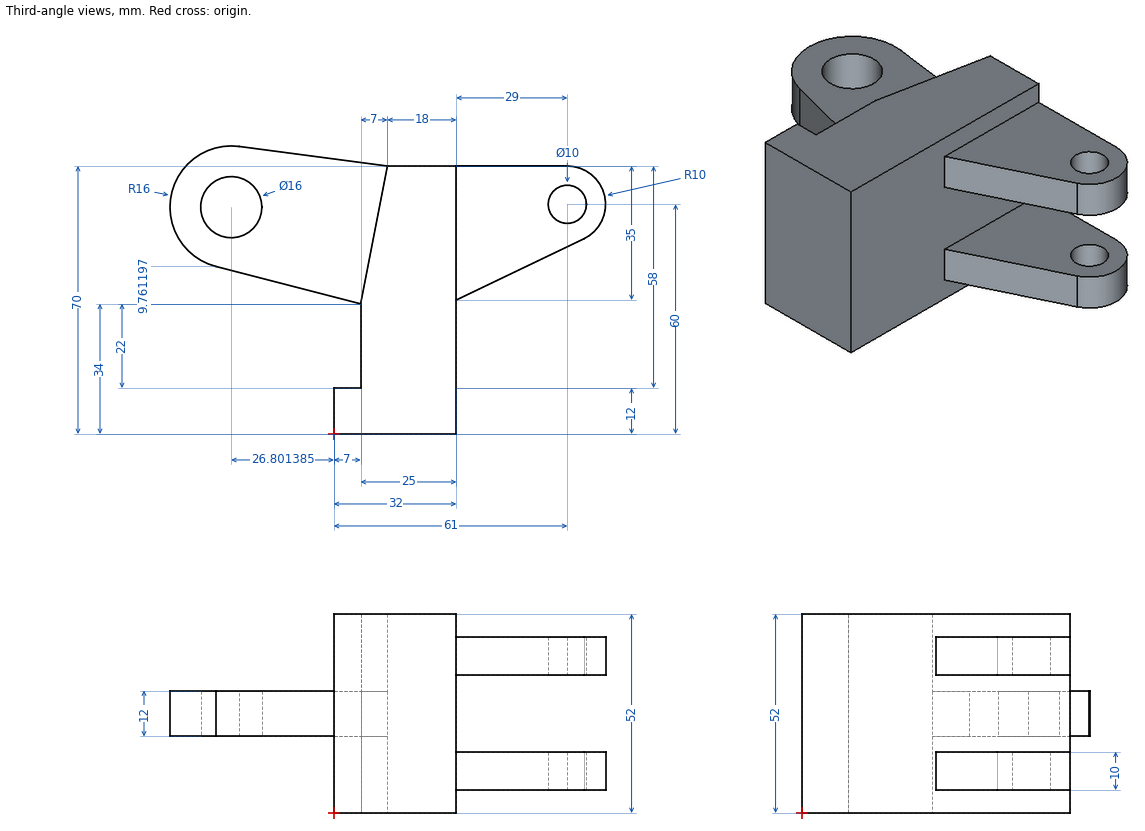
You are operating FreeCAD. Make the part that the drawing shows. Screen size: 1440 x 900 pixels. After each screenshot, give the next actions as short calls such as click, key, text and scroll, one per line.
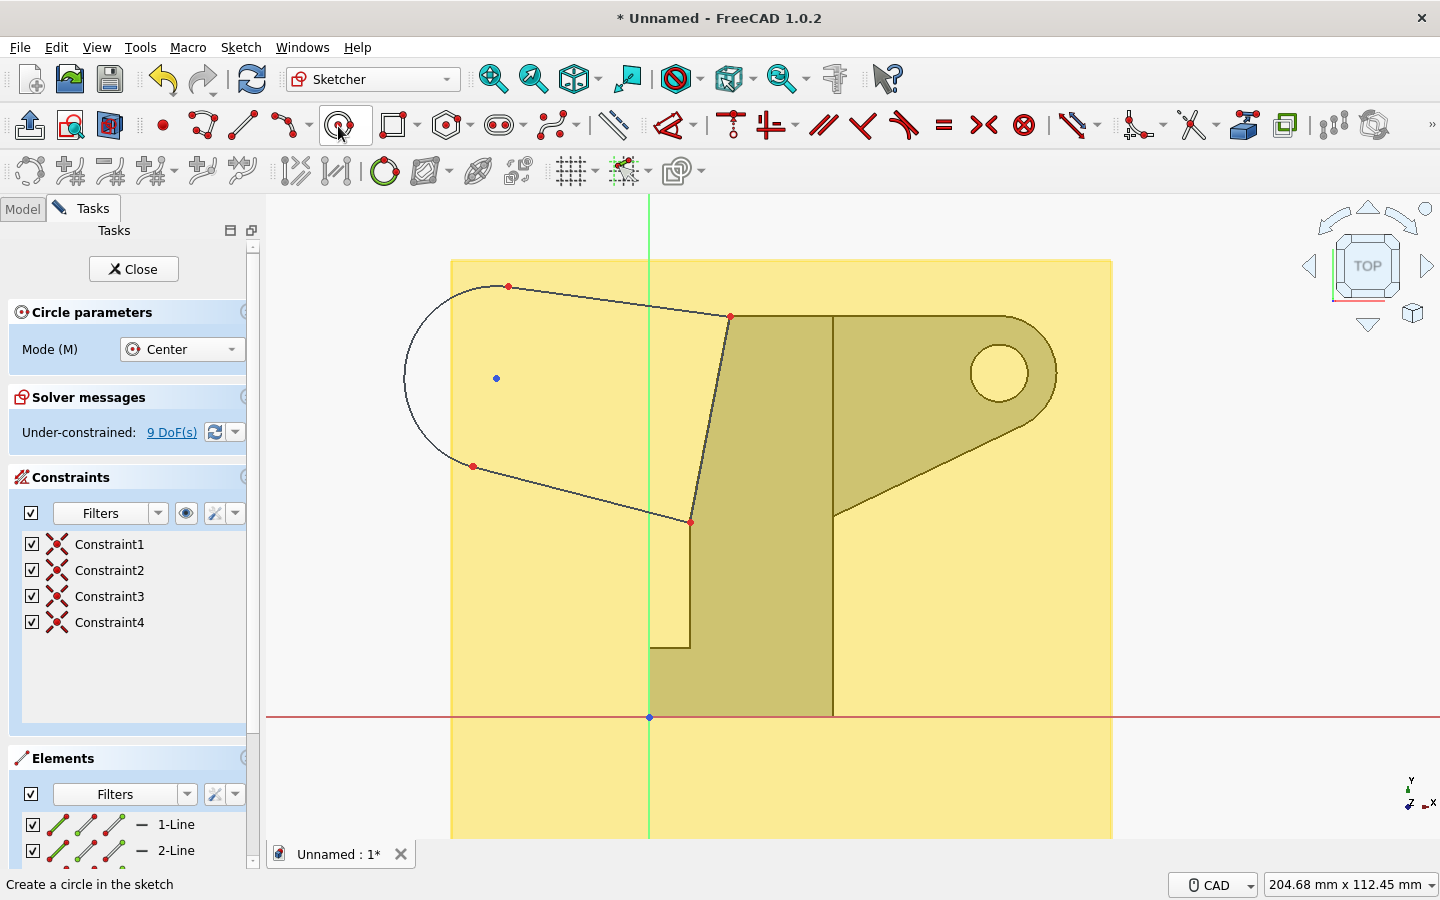
click(496, 377)
move(528, 345)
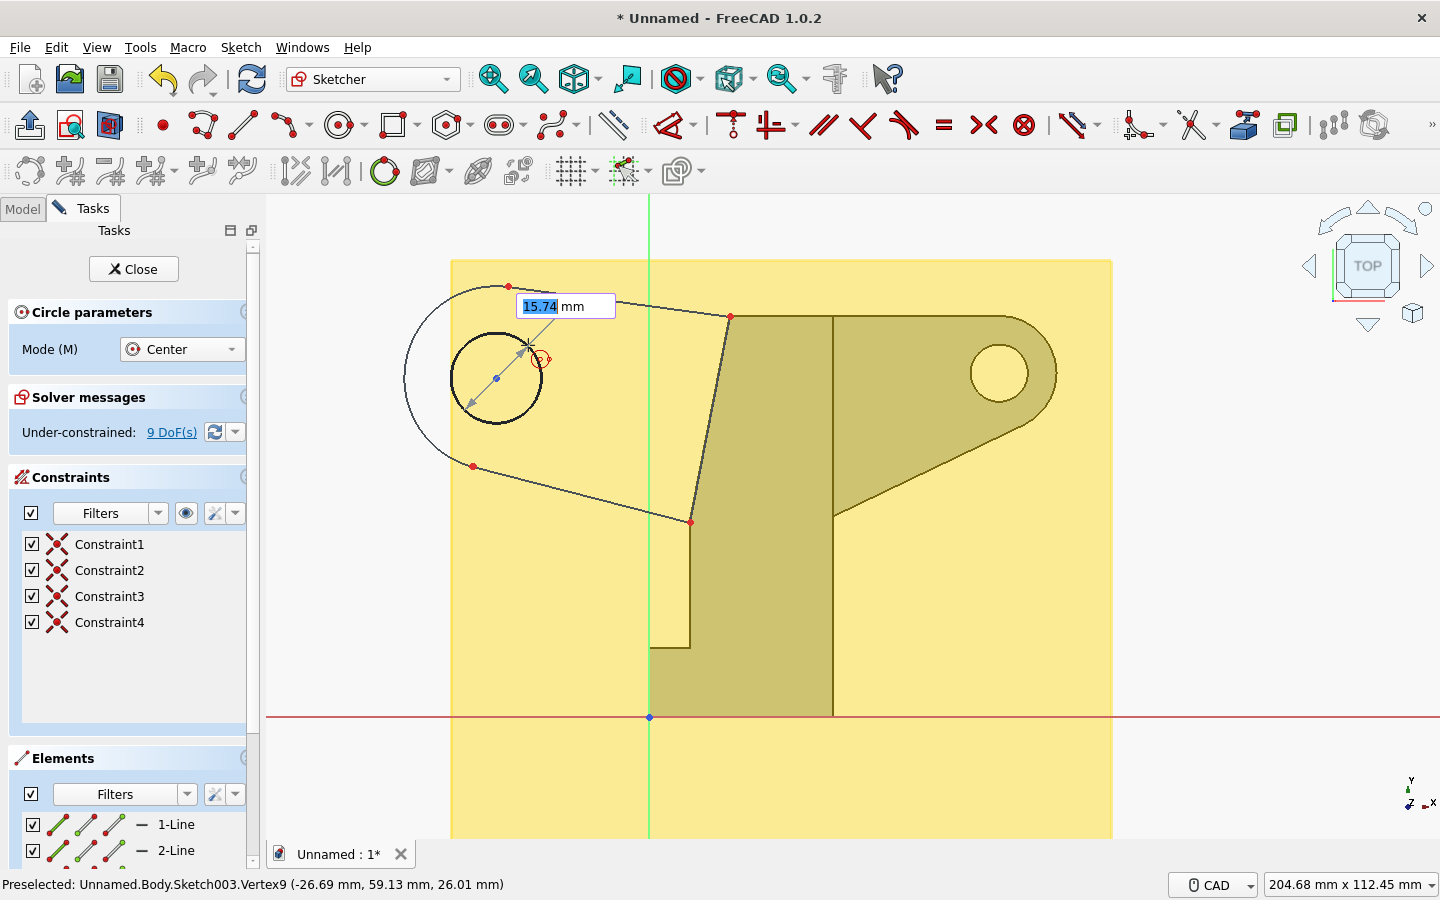
text(16)
key(Return)
key(Escape)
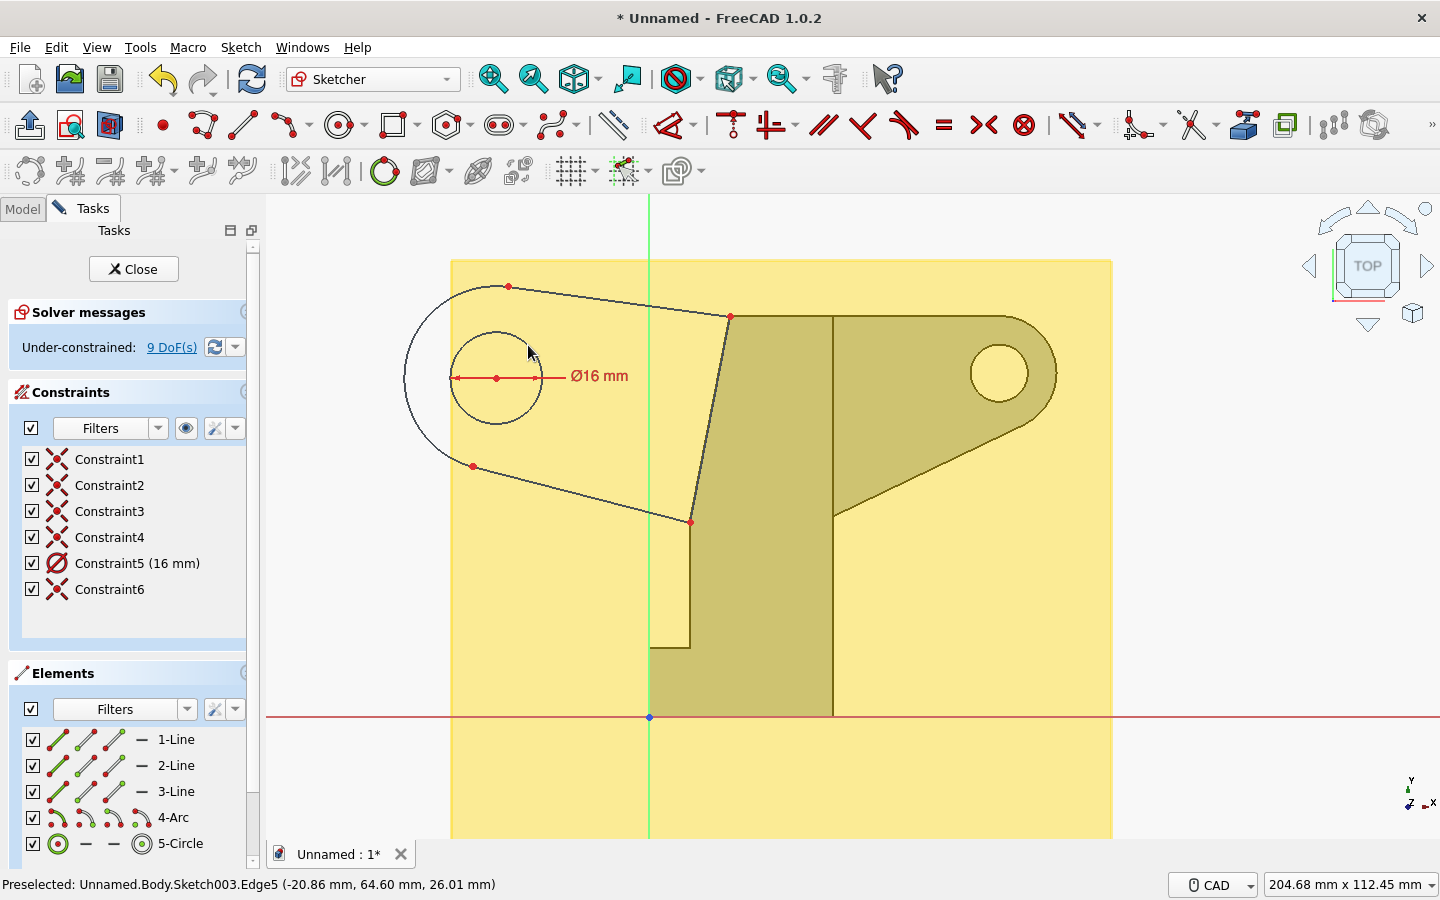
click(538, 484)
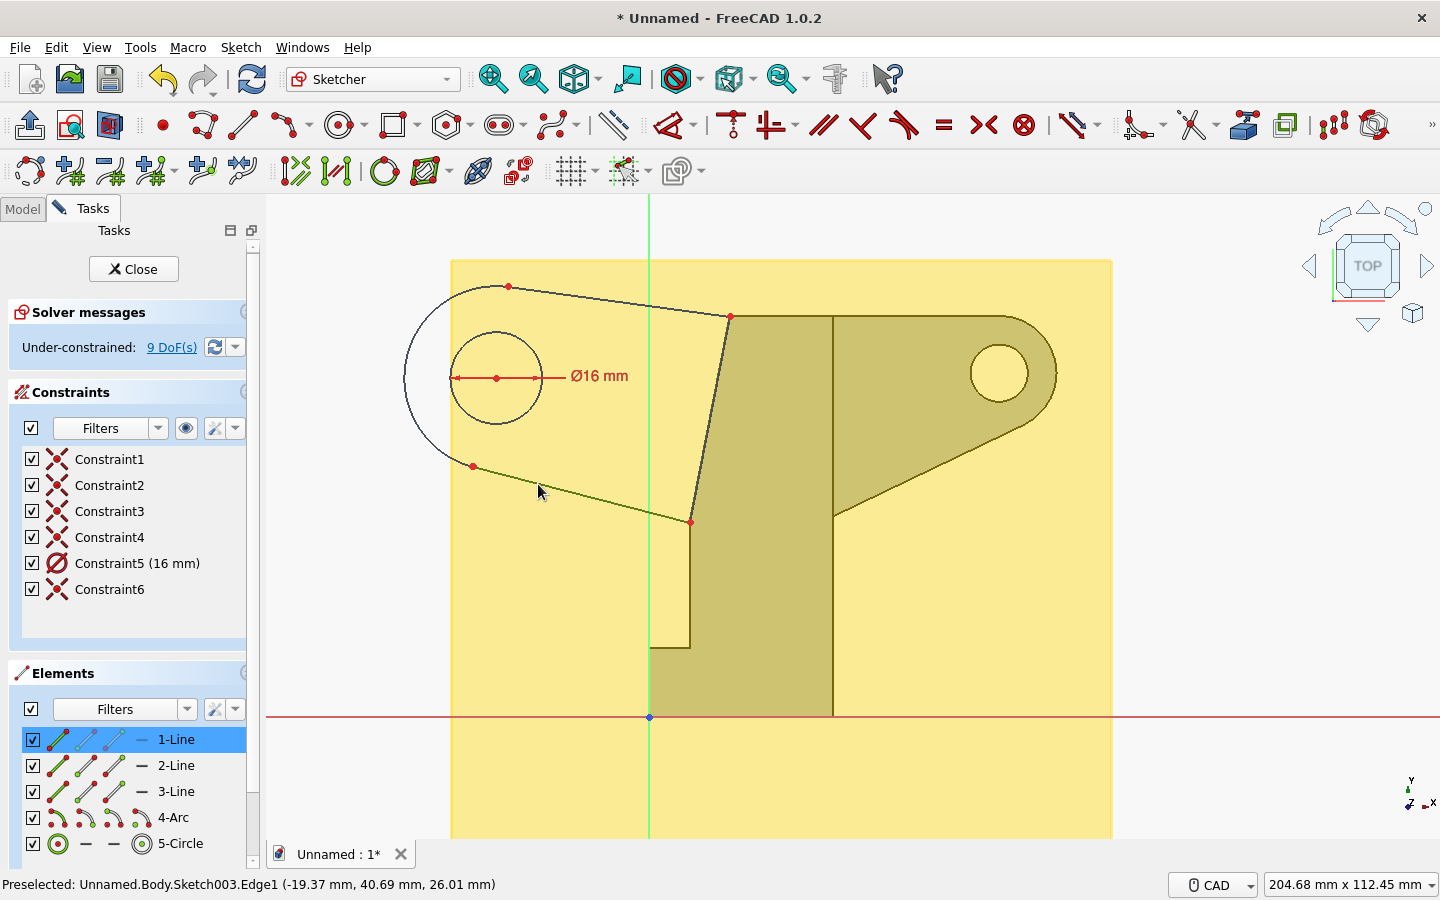
click(432, 313)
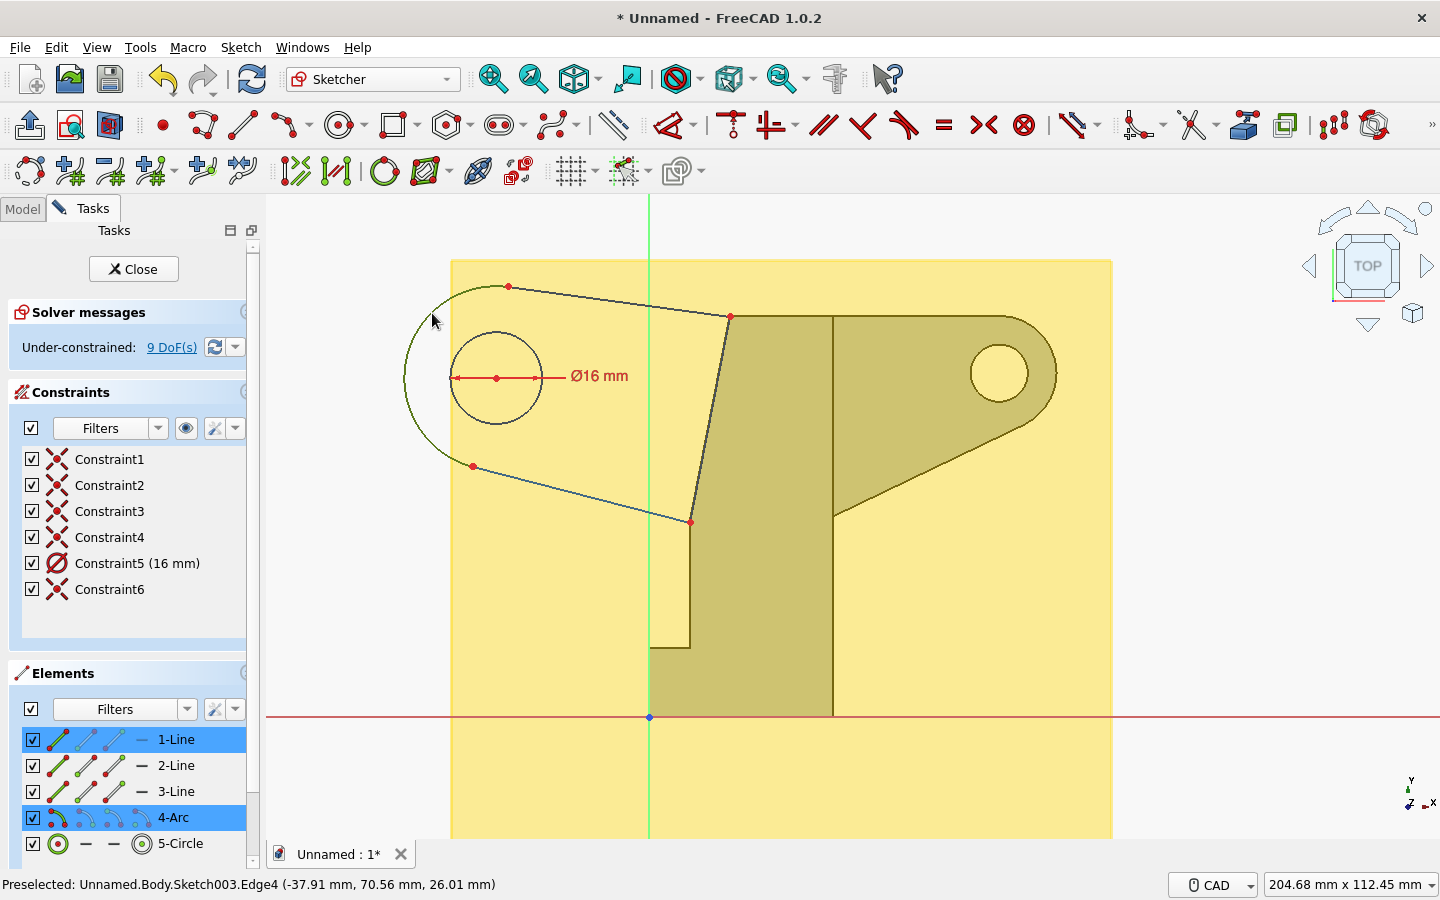
click(904, 126)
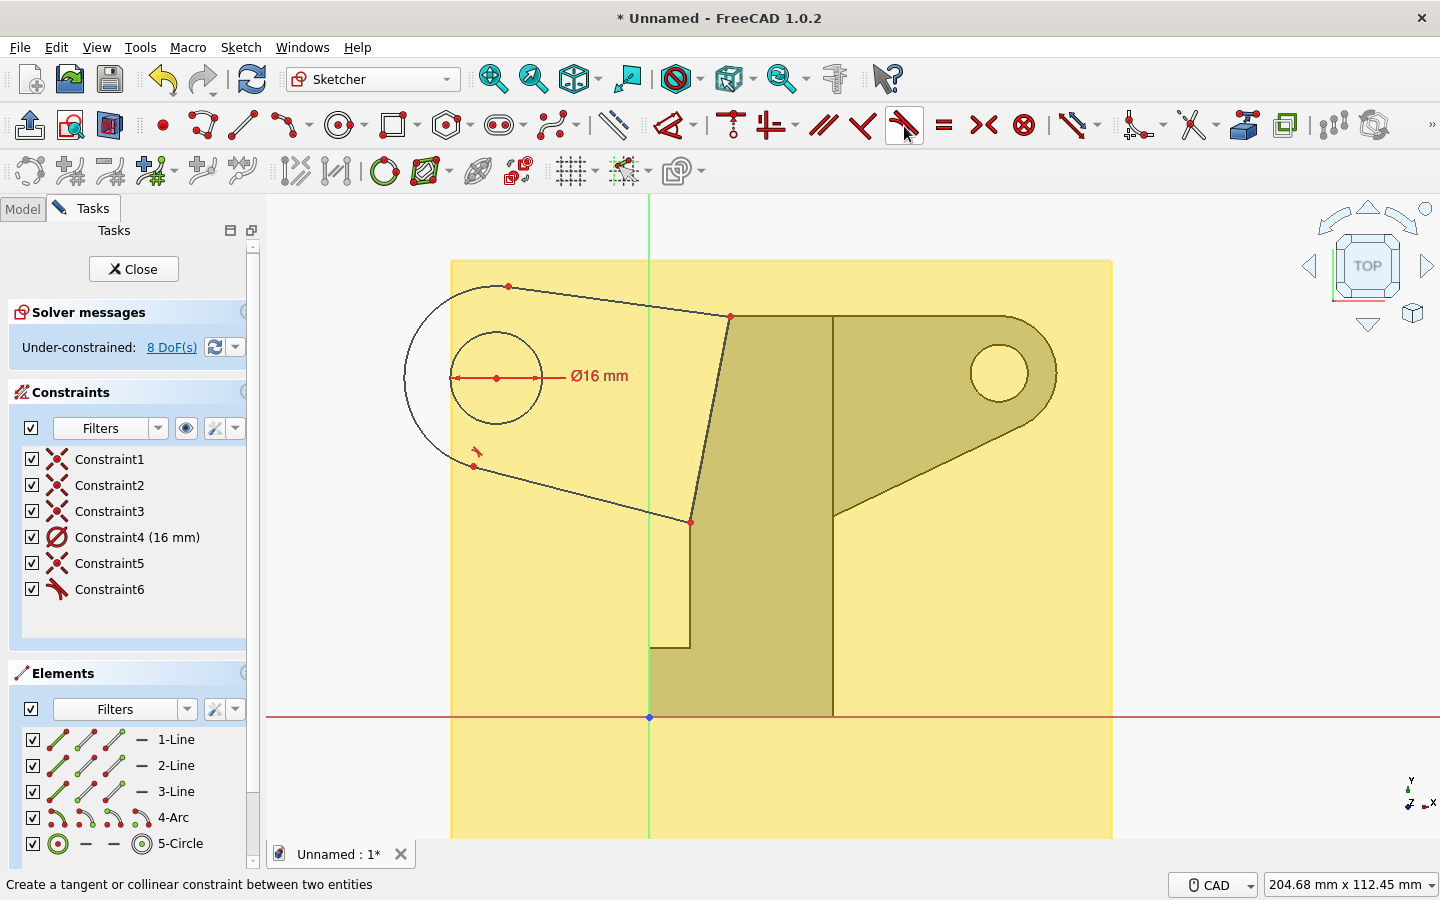
click(663, 308)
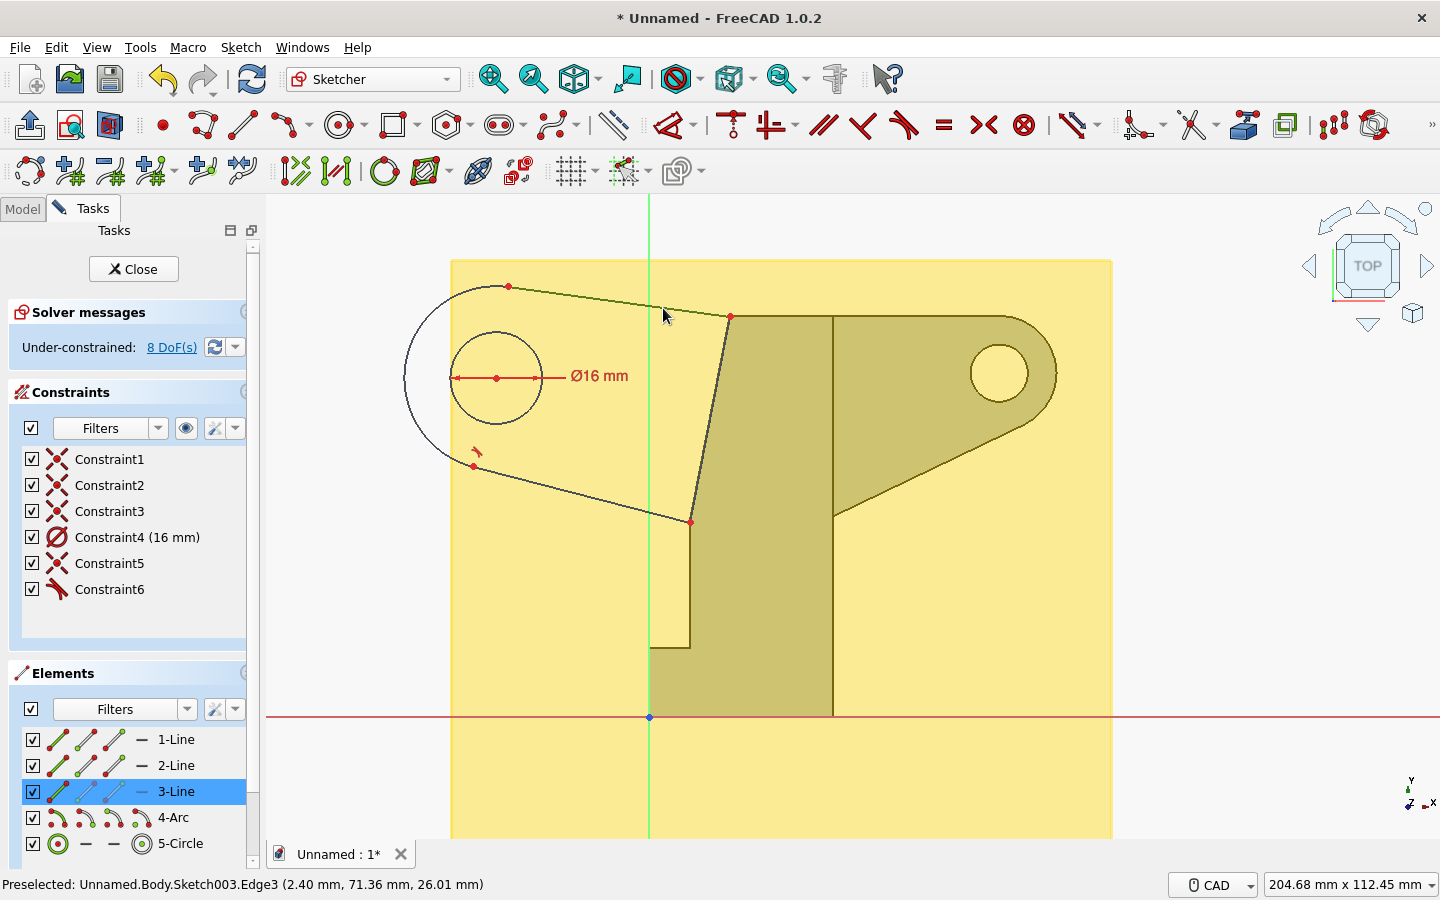
click(432, 313)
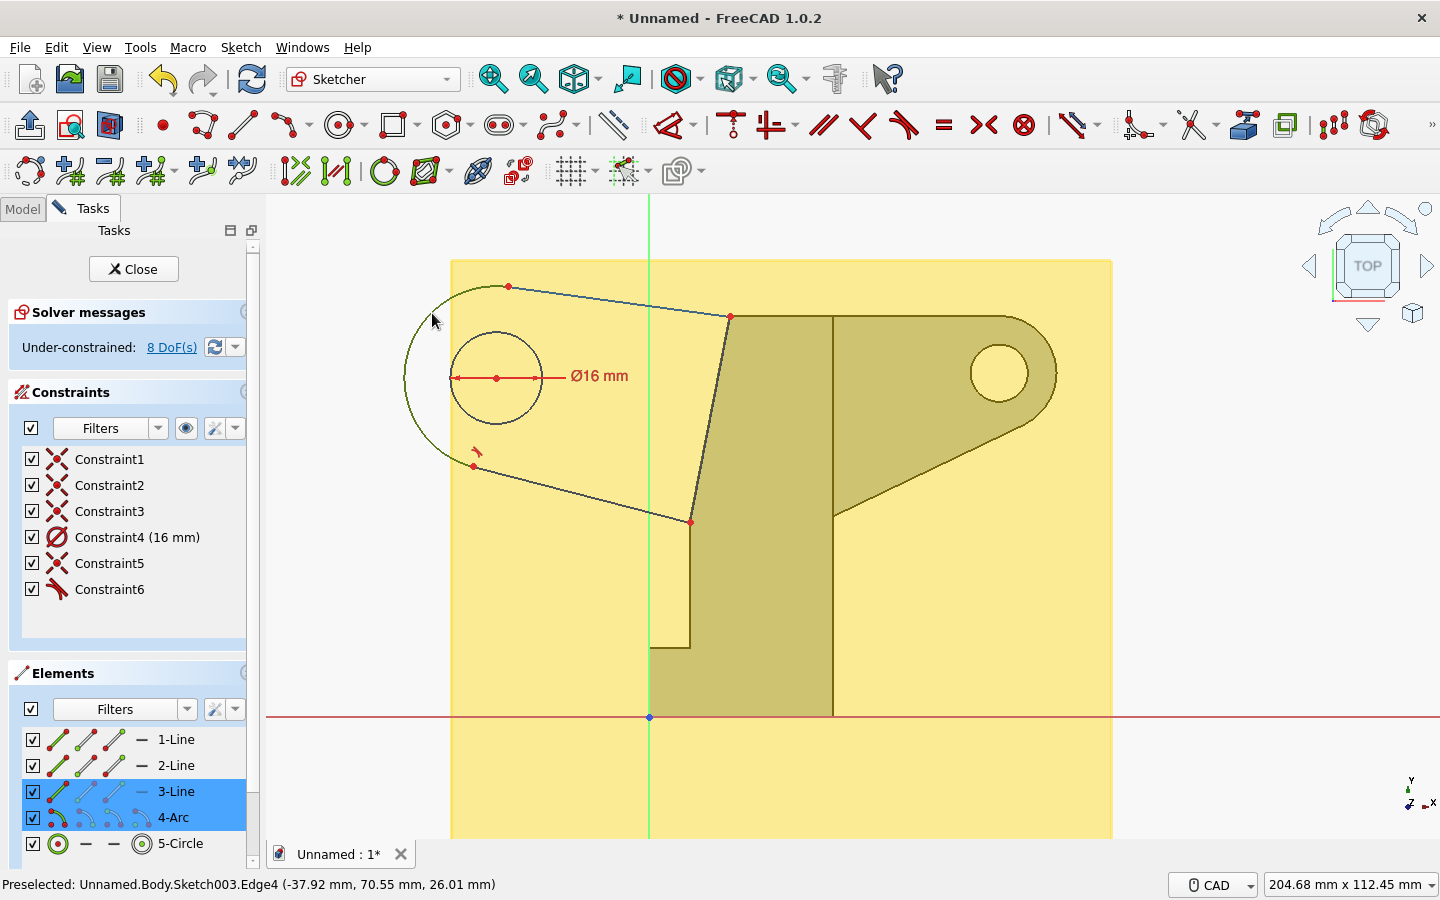
click(904, 126)